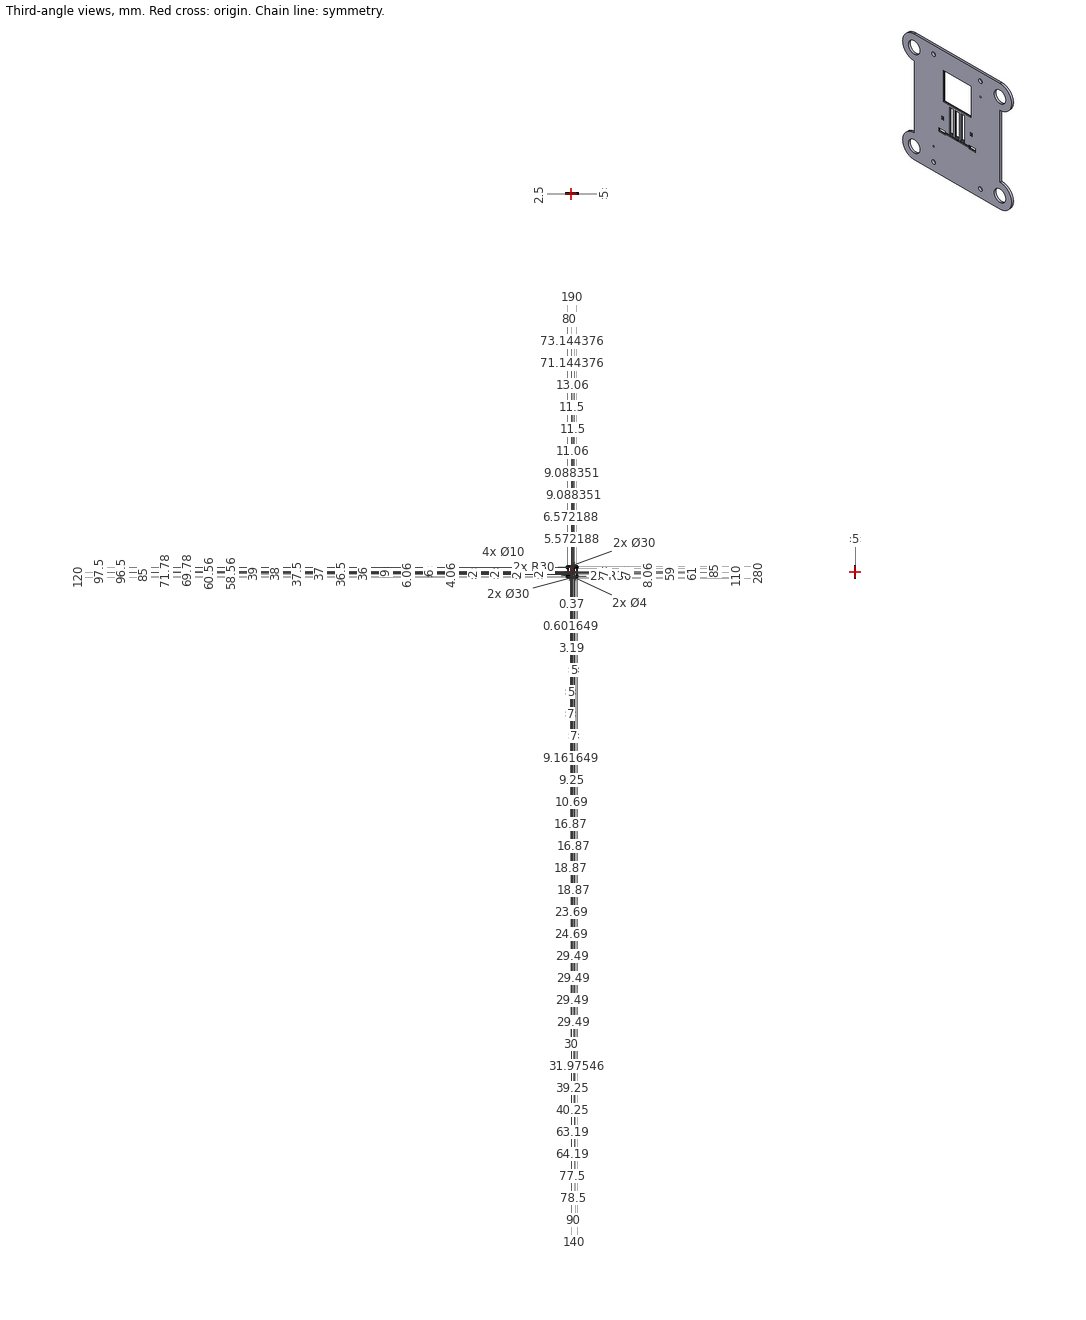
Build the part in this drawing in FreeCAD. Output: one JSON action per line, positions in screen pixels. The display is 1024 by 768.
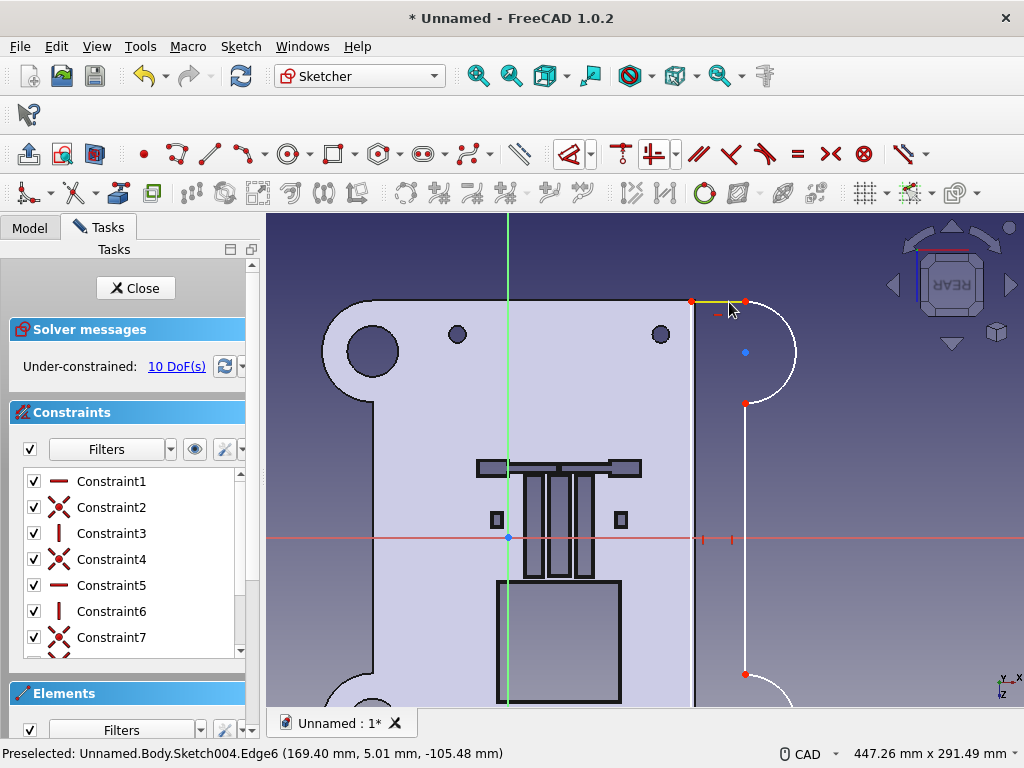
{"action": "left_click", "coordinate": [729, 302]}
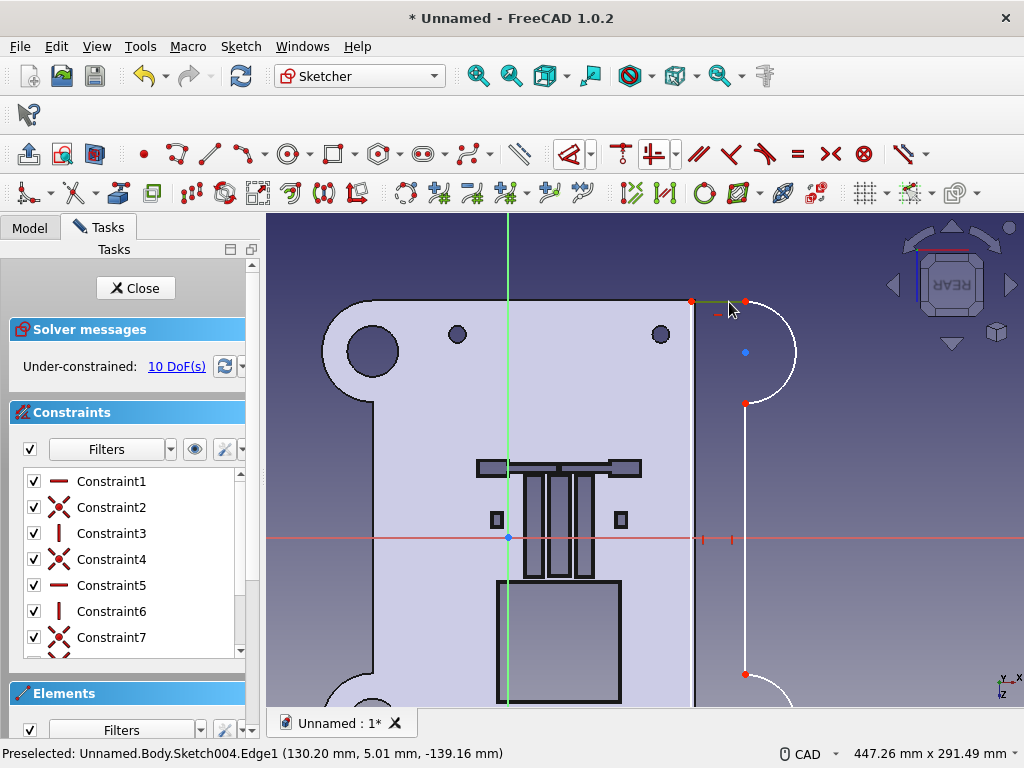
{"action": "left_click", "coordinate": [786, 382]}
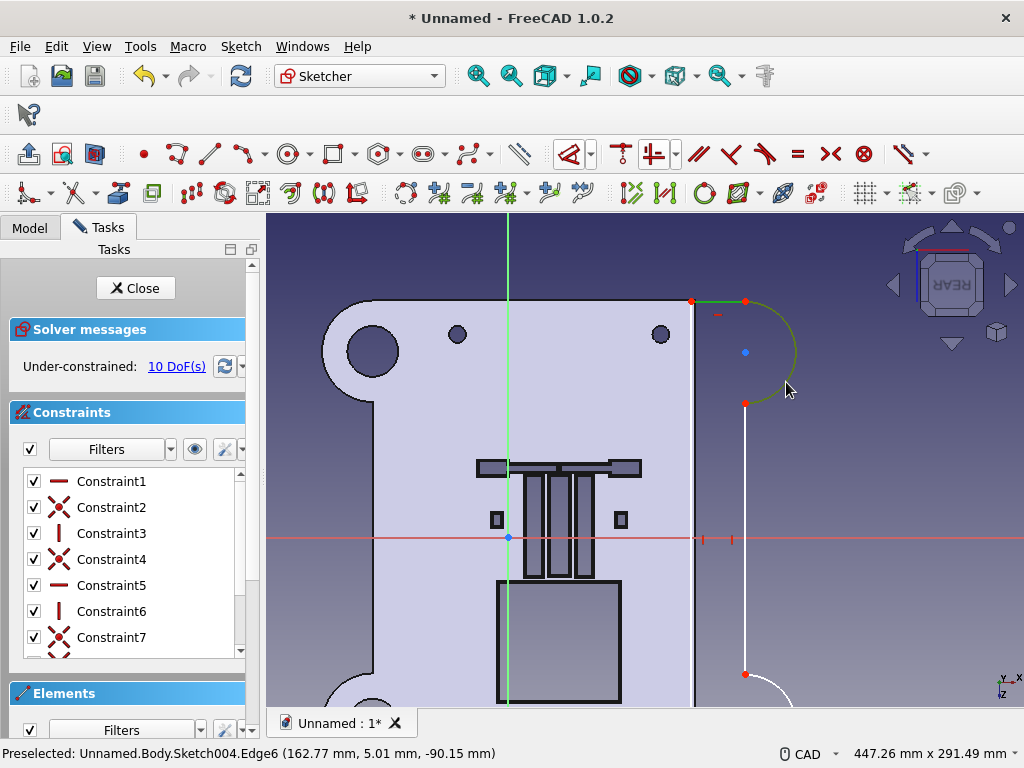
{"action": "key", "text": "t"}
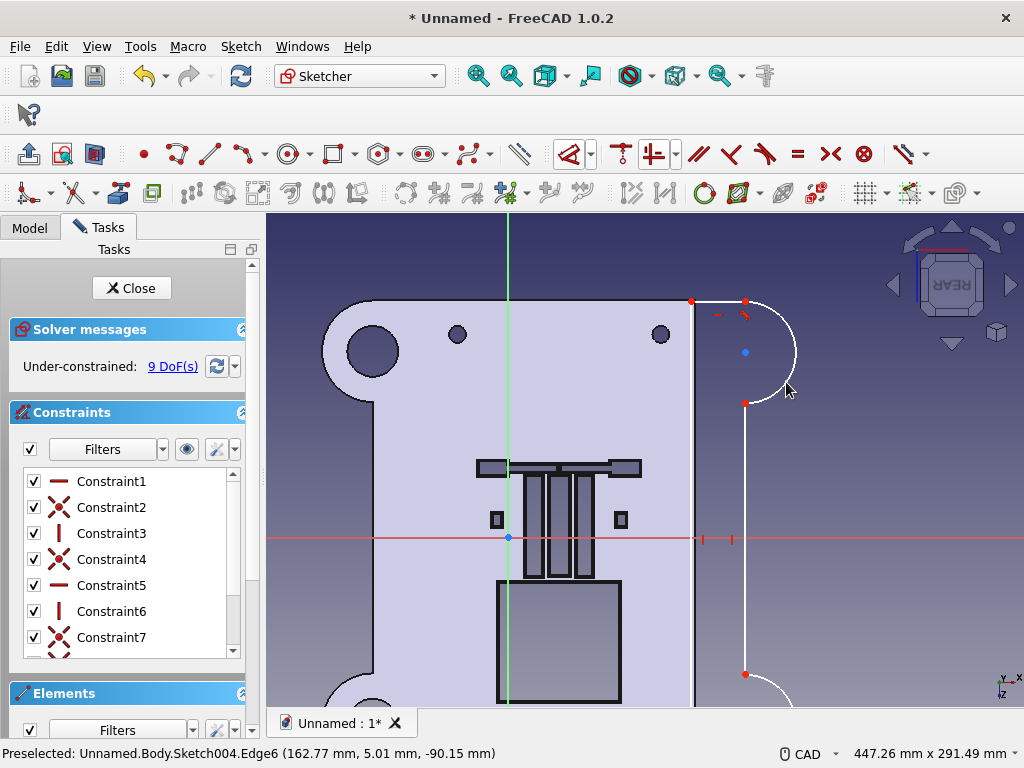
{"action": "scroll", "coordinate": [422, 302], "scroll_direction": "down", "scroll_amount": 2}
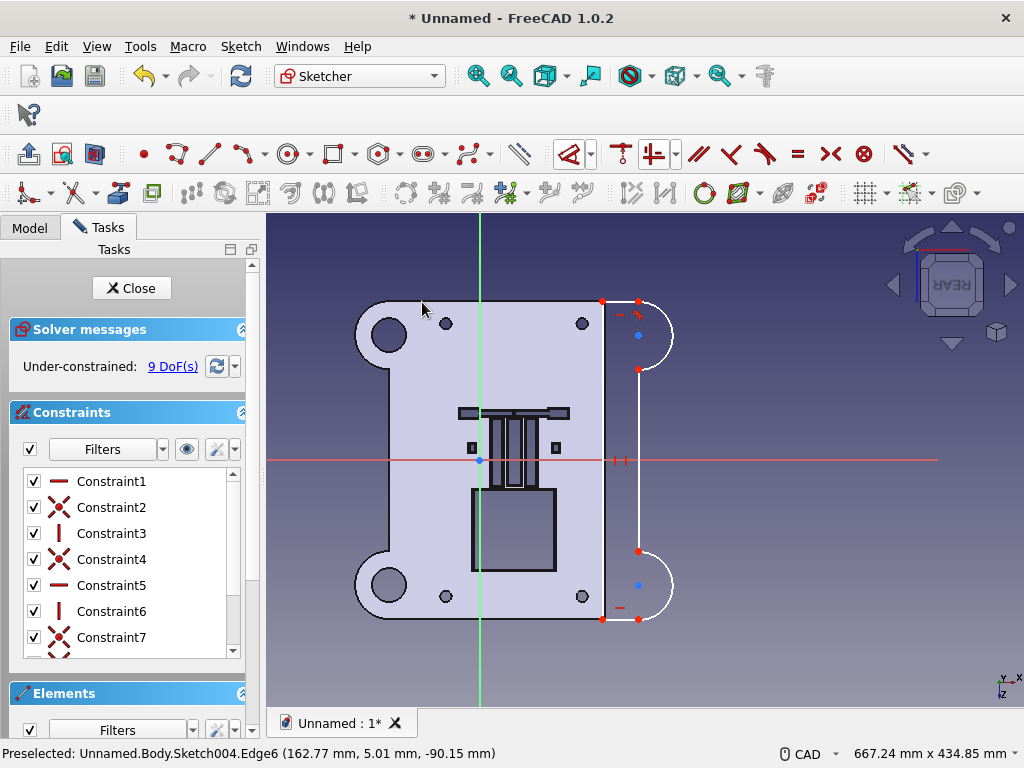
{"action": "scroll", "coordinate": [613, 620], "scroll_direction": "up", "scroll_amount": 2}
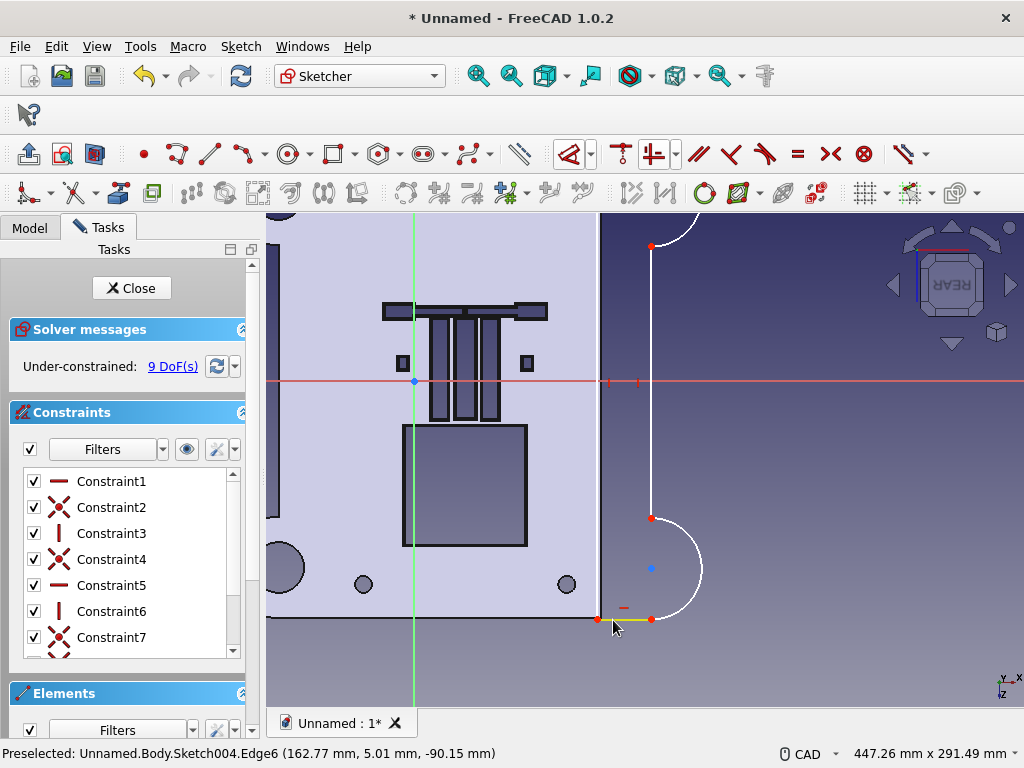
{"action": "left_click", "coordinate": [613, 620]}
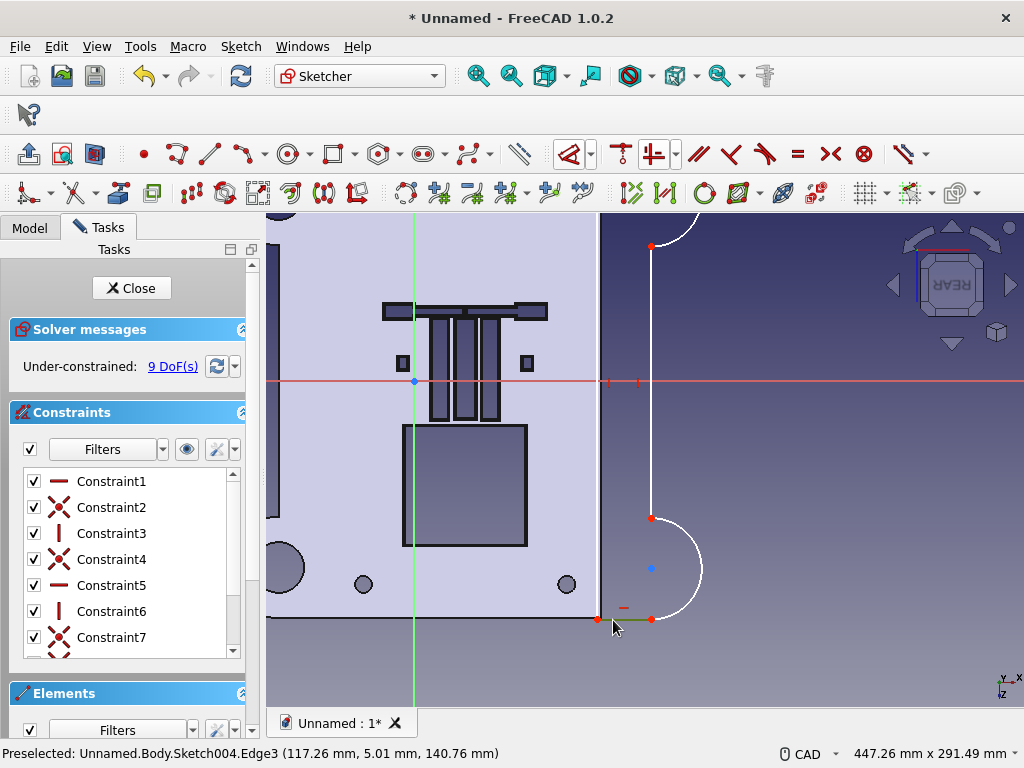
{"action": "left_click", "coordinate": [692, 599]}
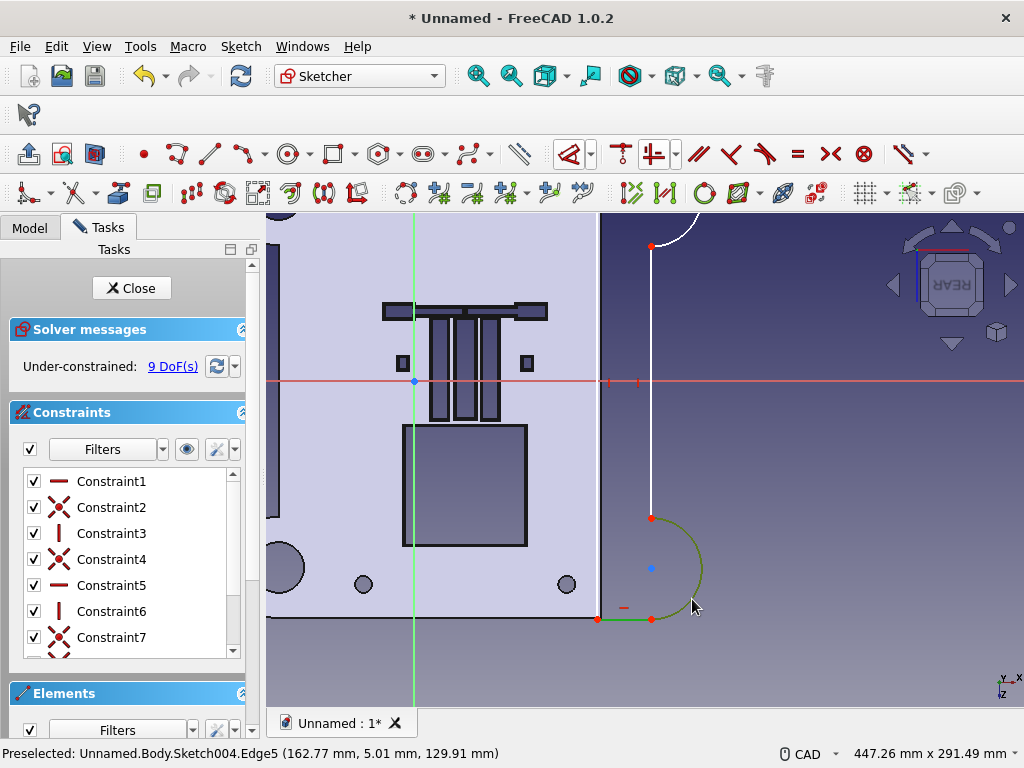
{"action": "left_click", "coordinate": [765, 154]}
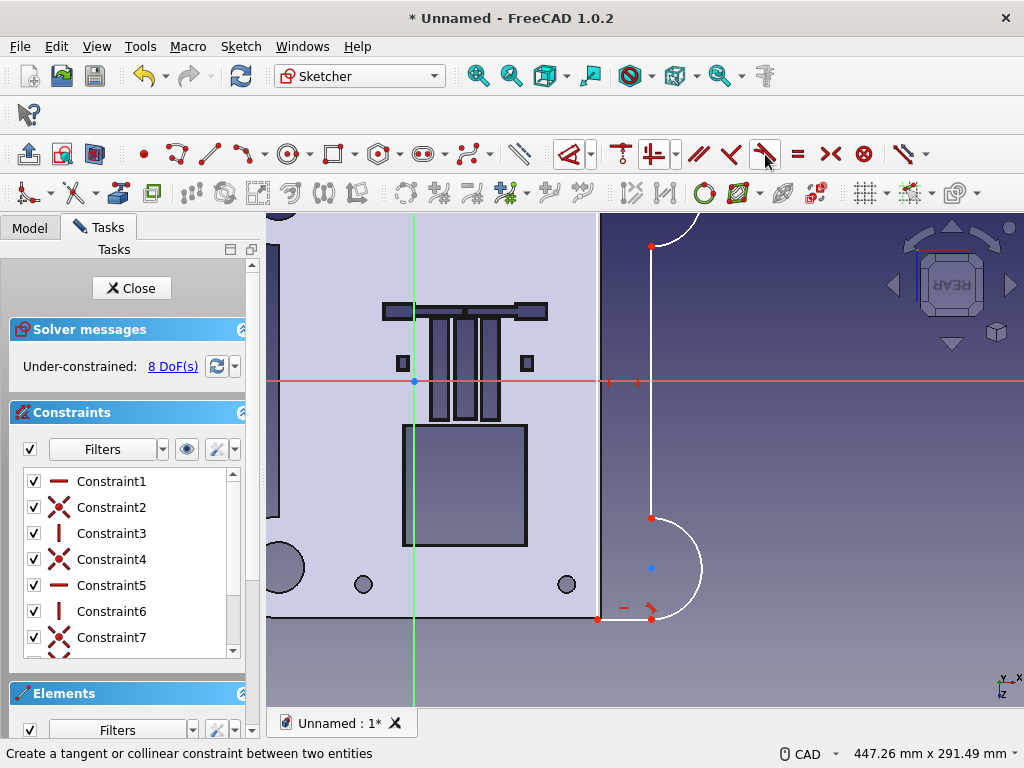
{"action": "left_click", "coordinate": [692, 599]}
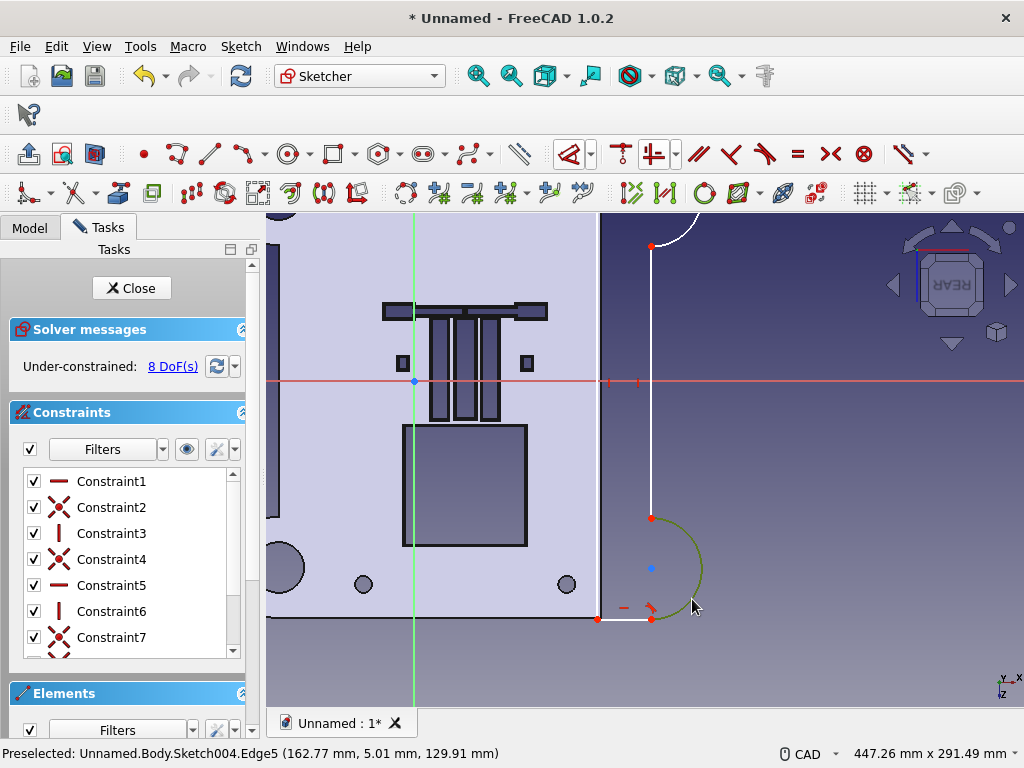
{"action": "scroll", "coordinate": [613, 621], "scroll_direction": "down", "scroll_amount": 2}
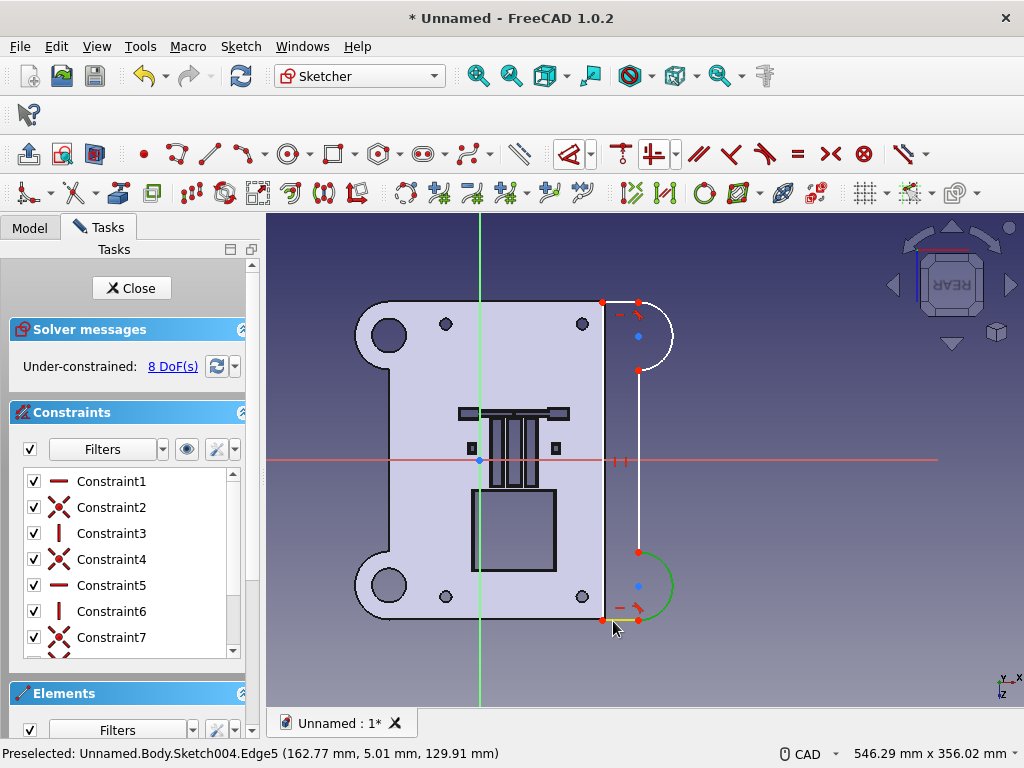
{"action": "left_click", "coordinate": [666, 356]}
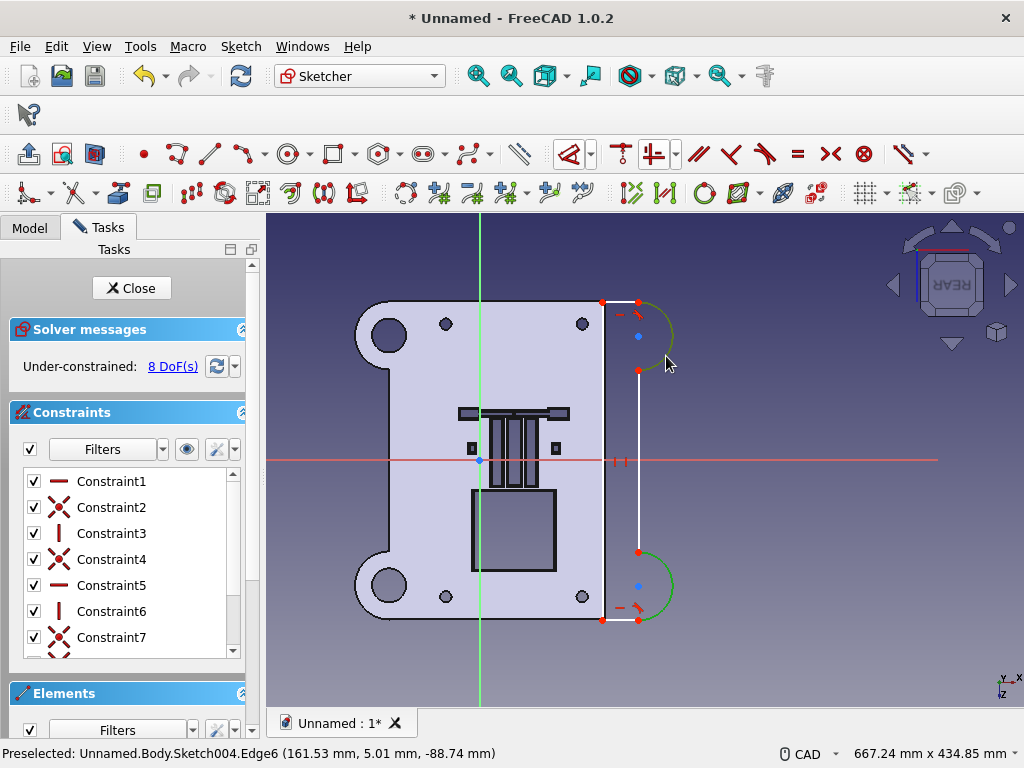
{"action": "key", "text": "e"}